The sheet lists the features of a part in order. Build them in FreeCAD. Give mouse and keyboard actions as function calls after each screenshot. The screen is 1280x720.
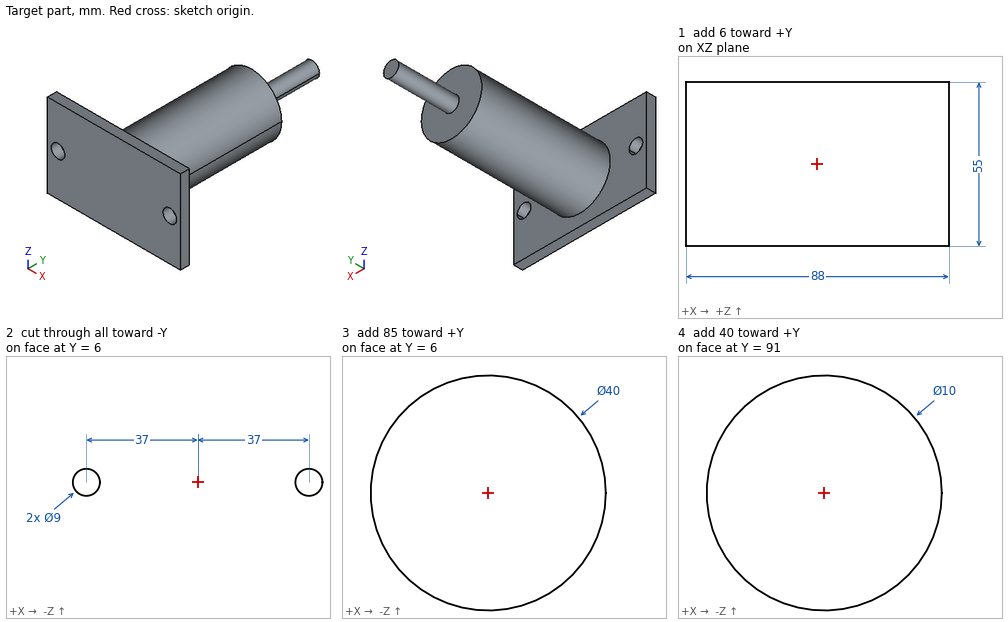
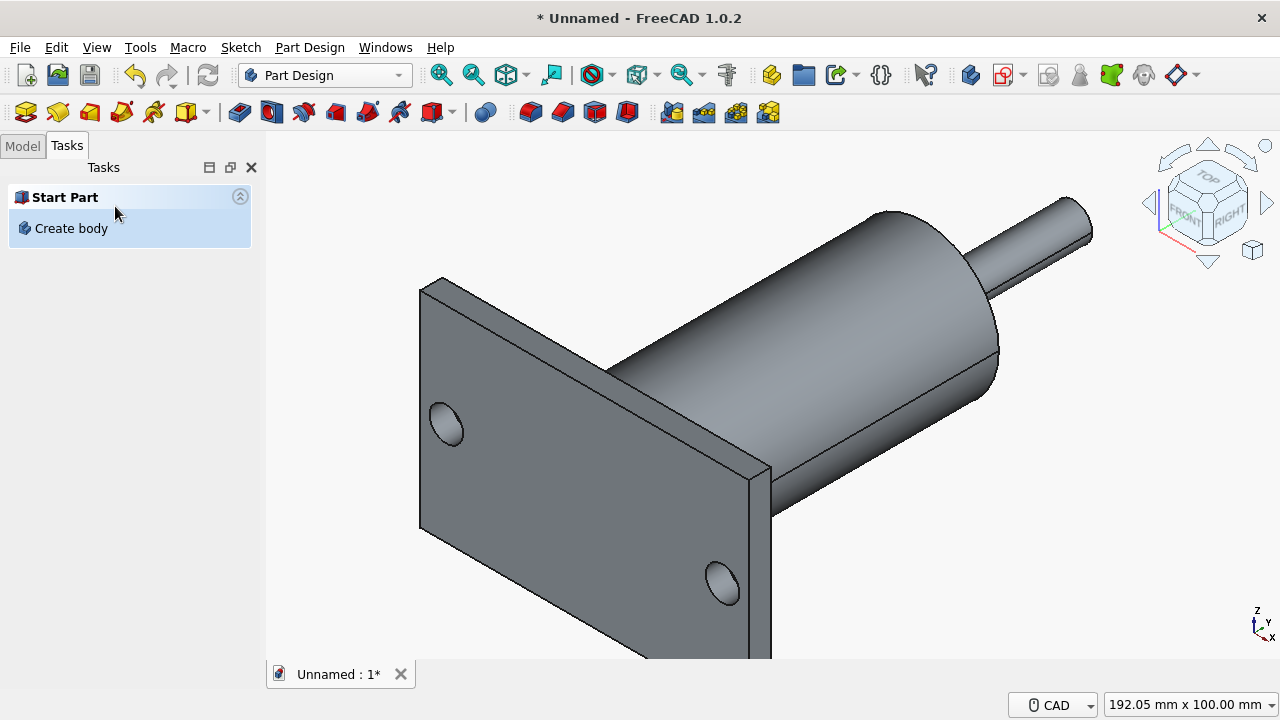
key(v)
key(f)